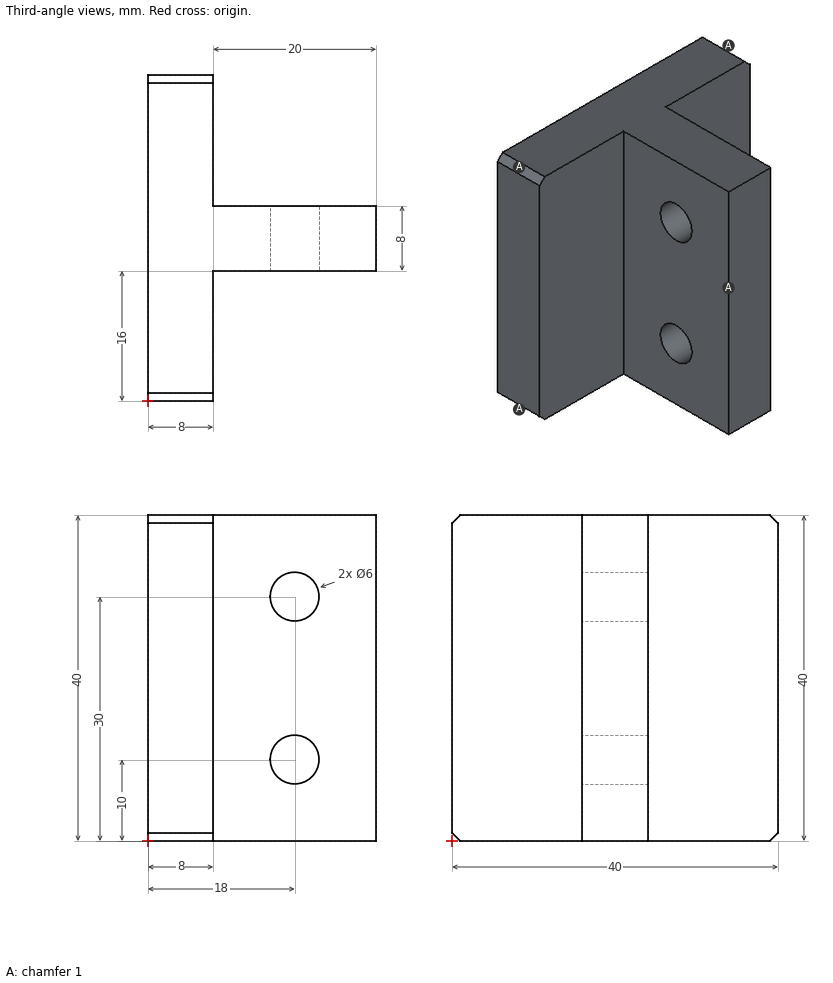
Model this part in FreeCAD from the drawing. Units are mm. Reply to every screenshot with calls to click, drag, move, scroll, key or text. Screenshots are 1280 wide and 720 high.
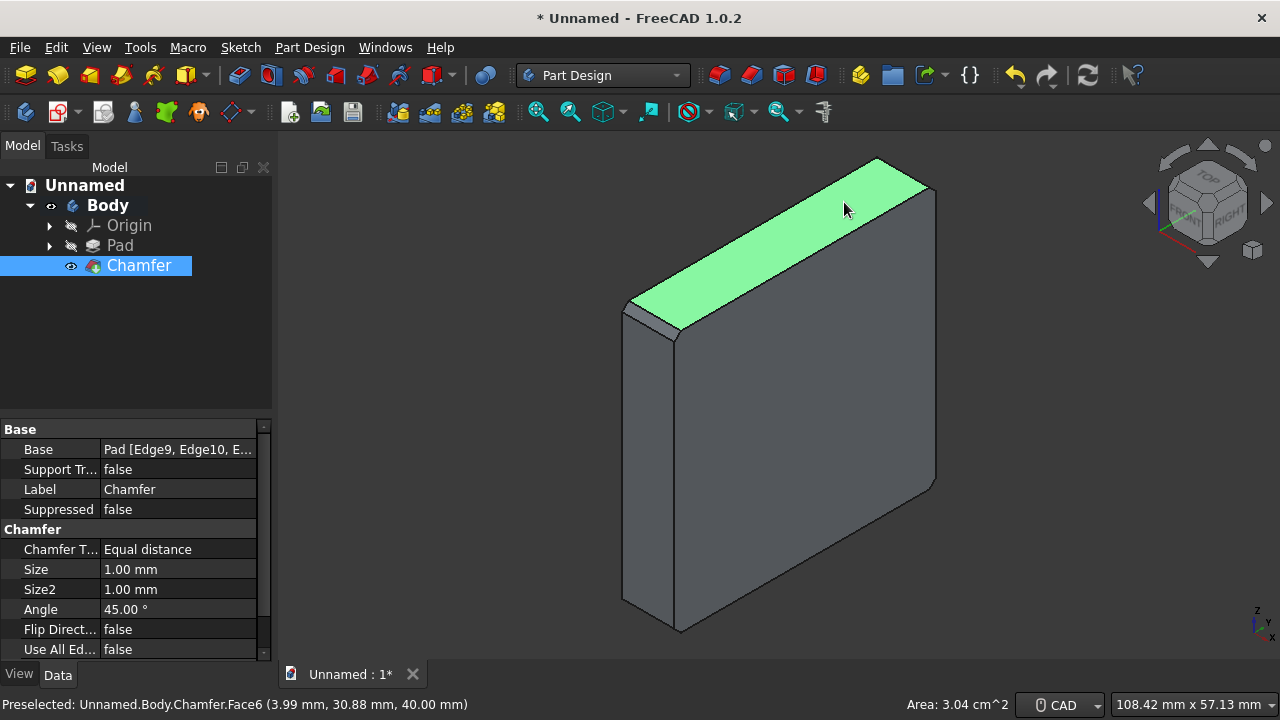
click(58, 112)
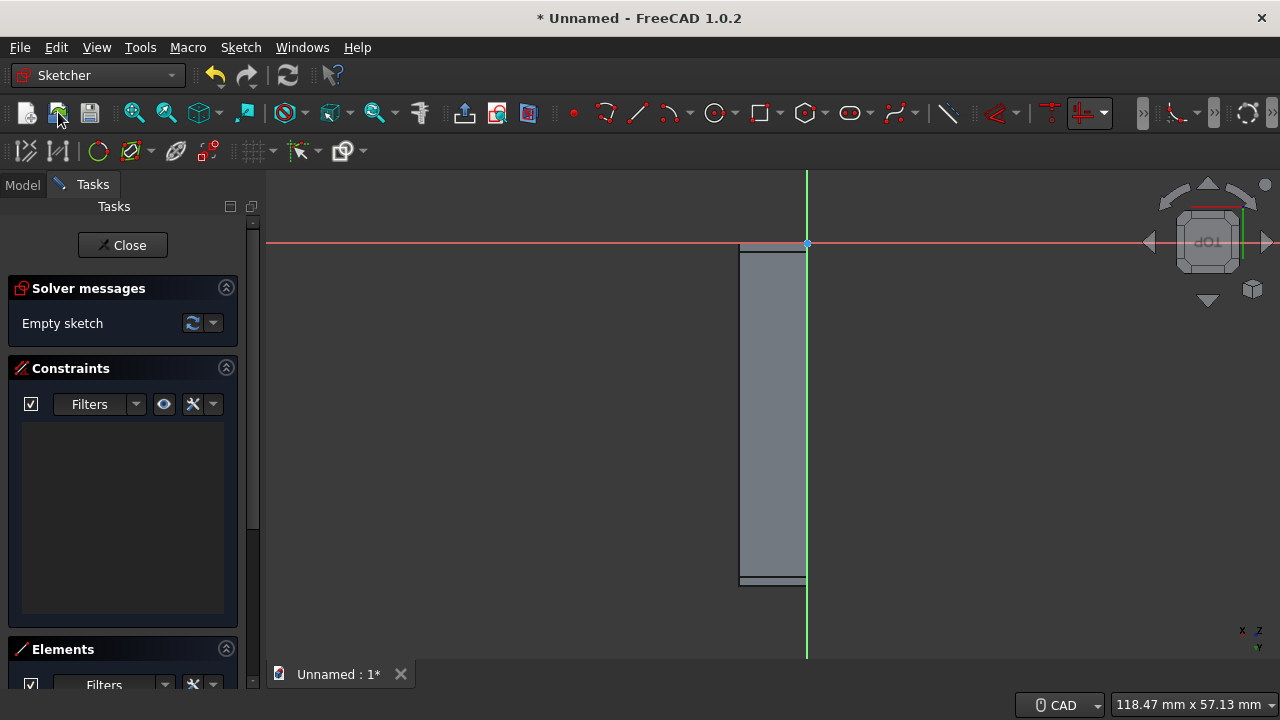
scroll(653, 207, up, 2)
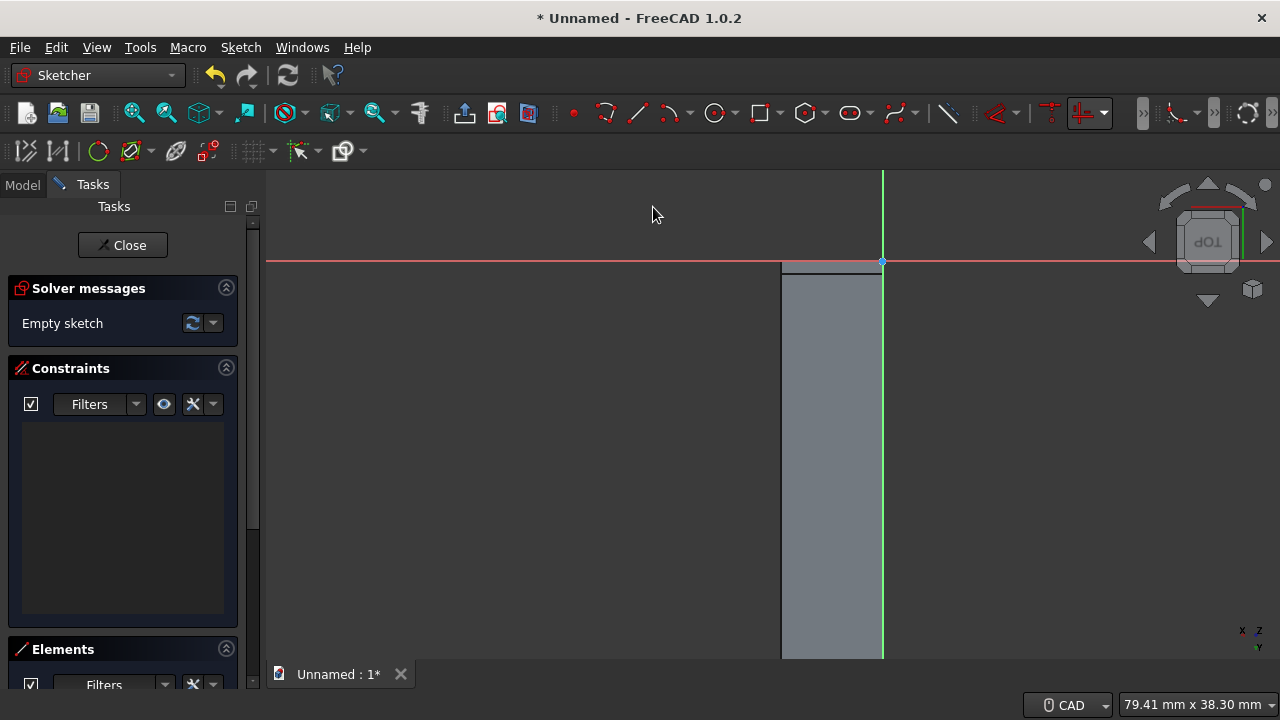
click(760, 114)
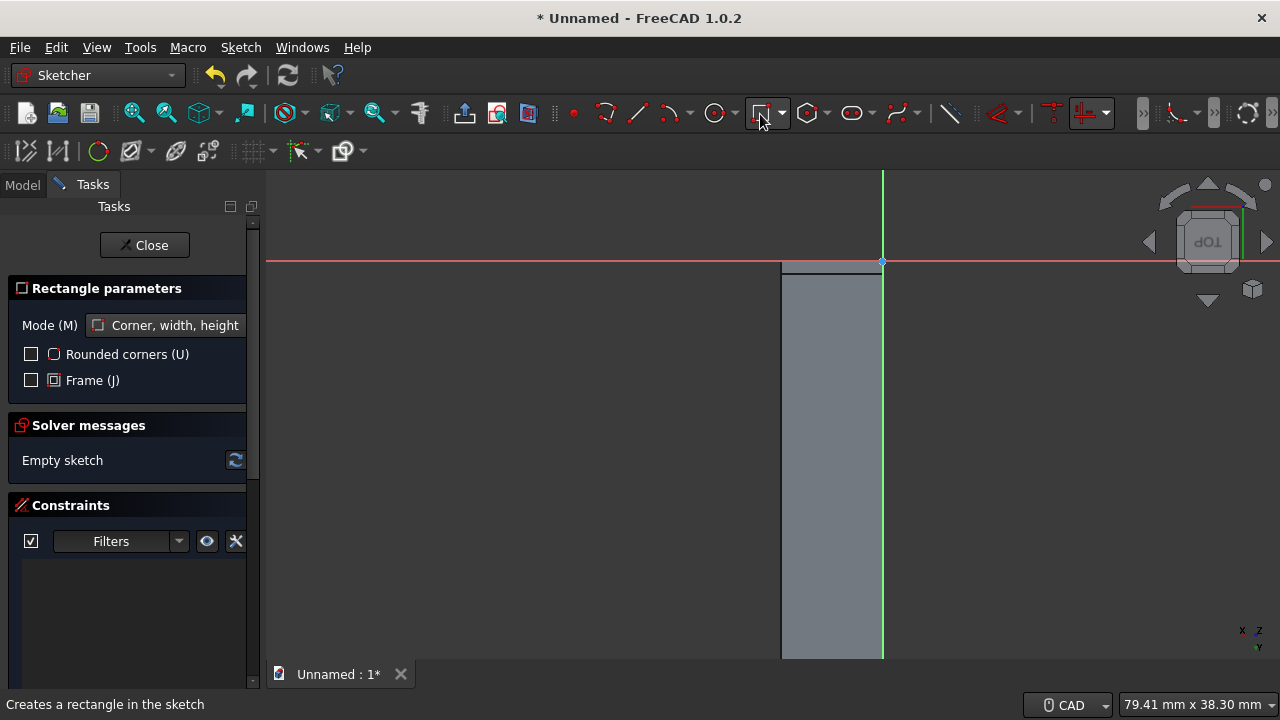
click(525, 465)
click(781, 568)
key(Escape)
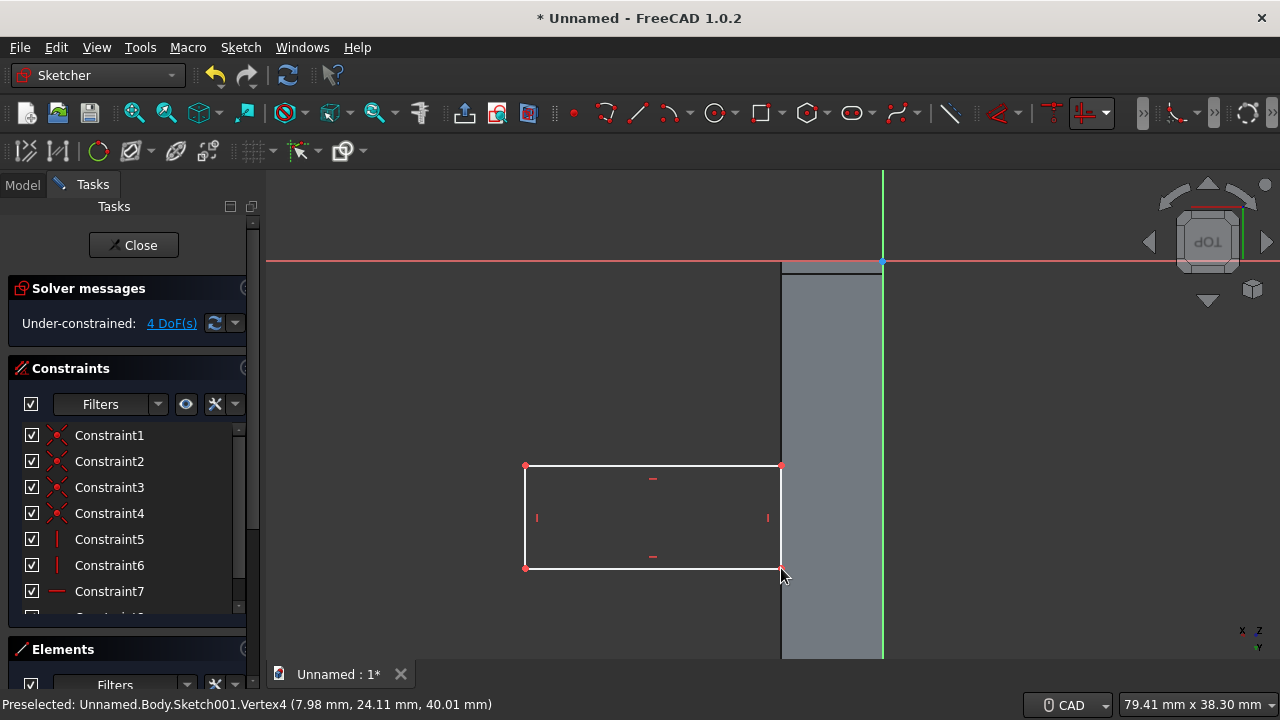
click(998, 114)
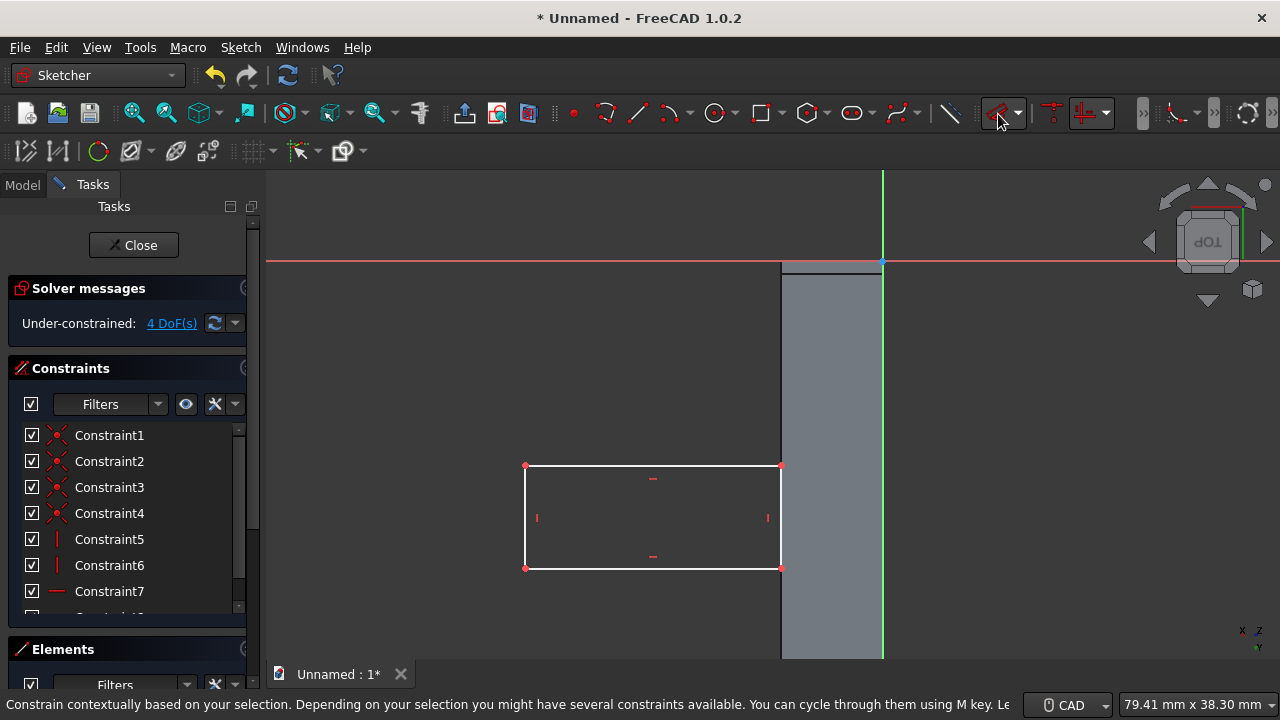
click(525, 497)
click(491, 518)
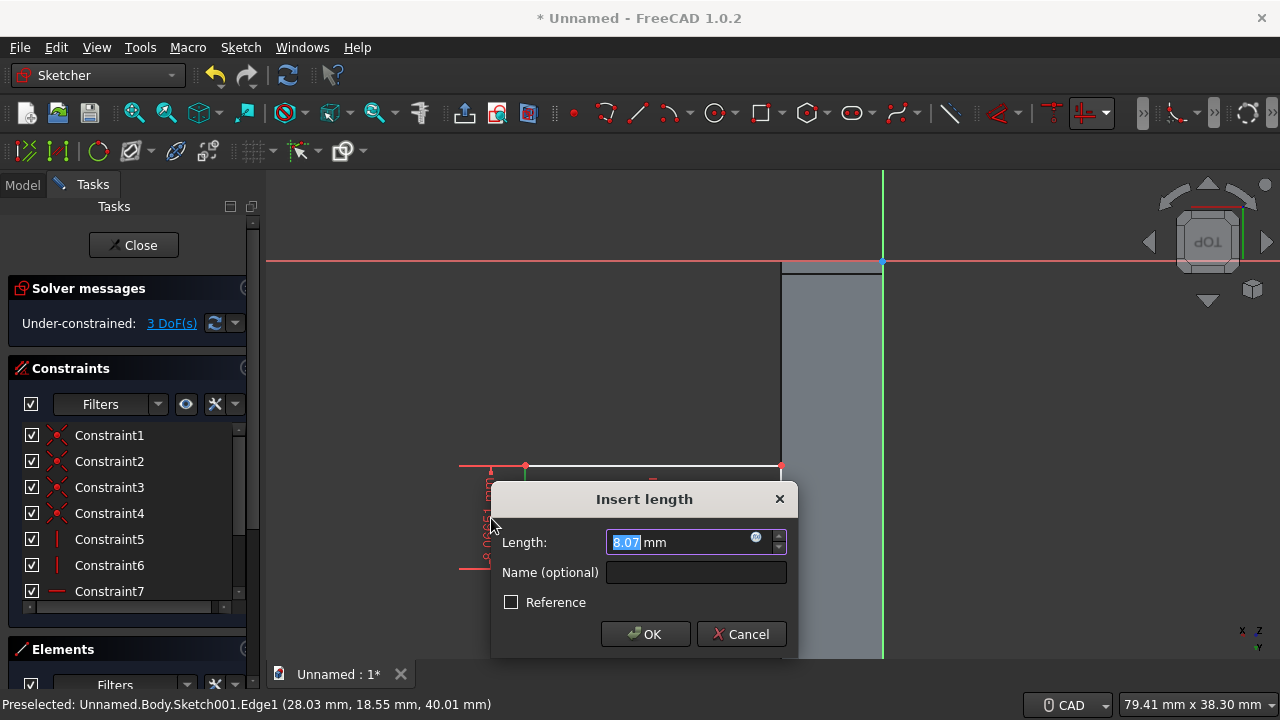
text(8)
key(Return)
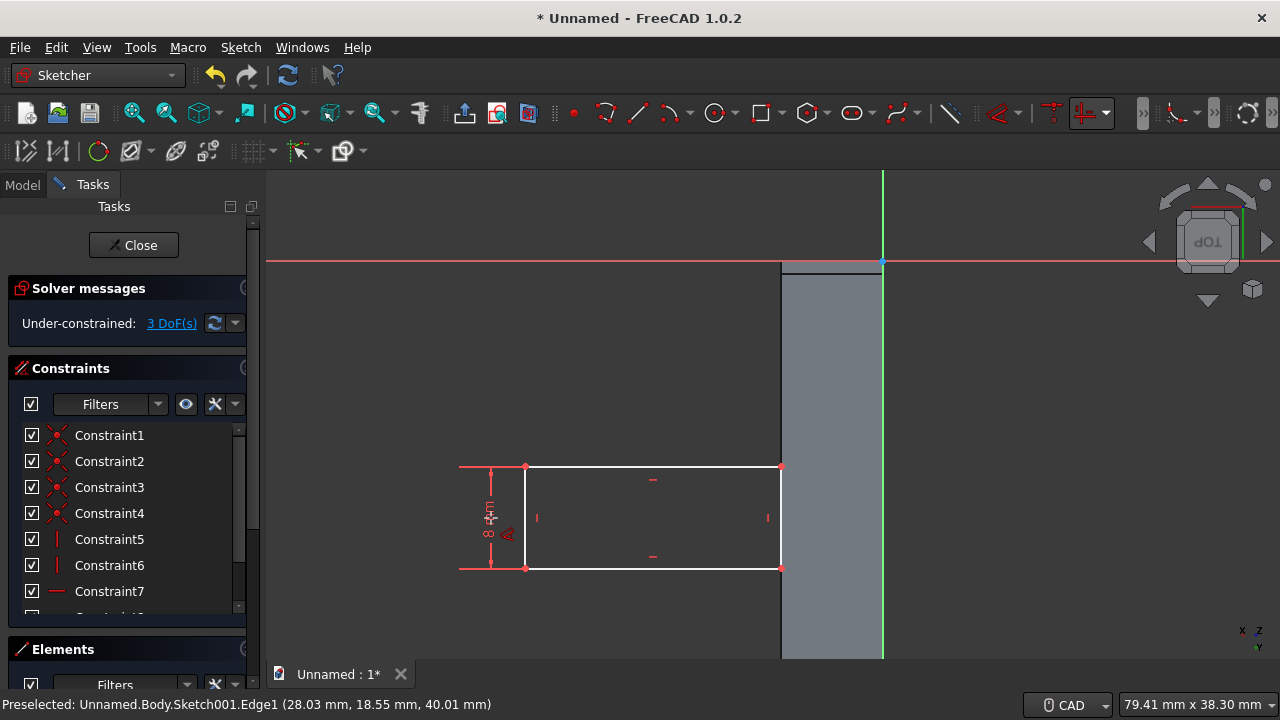
click(602, 569)
click(653, 603)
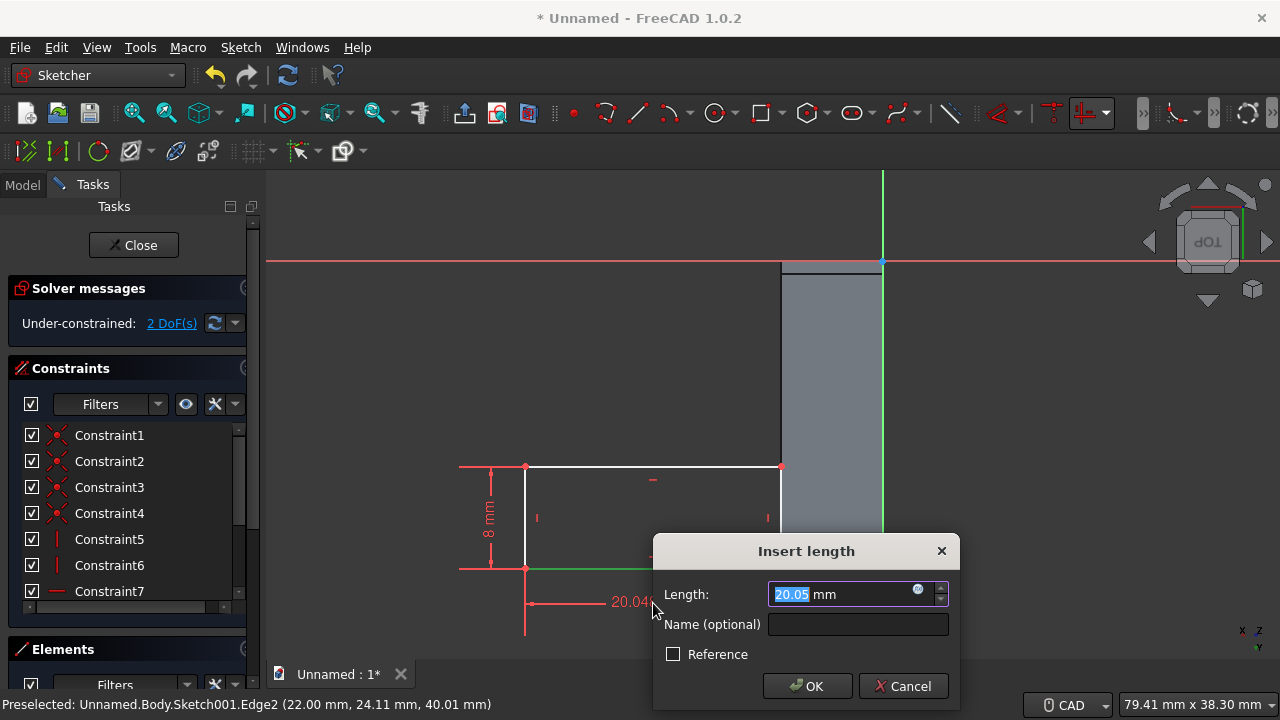
text(20)
key(Return)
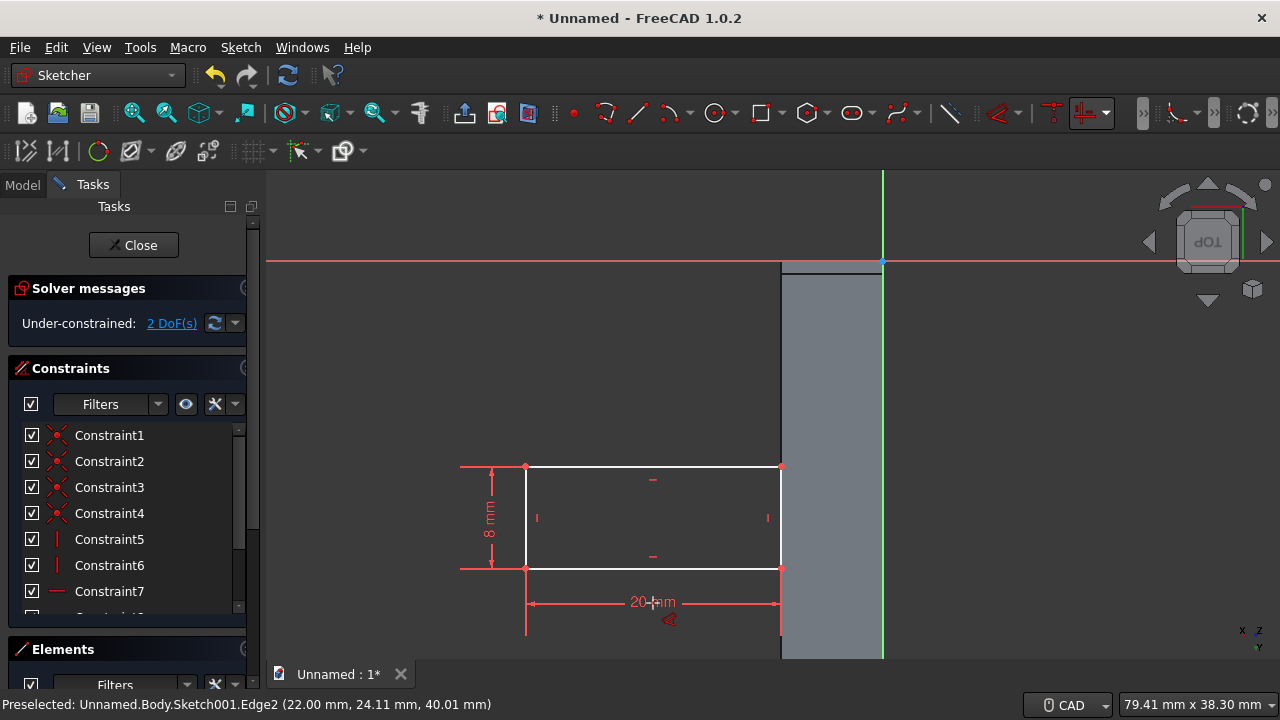
click(781, 569)
click(832, 603)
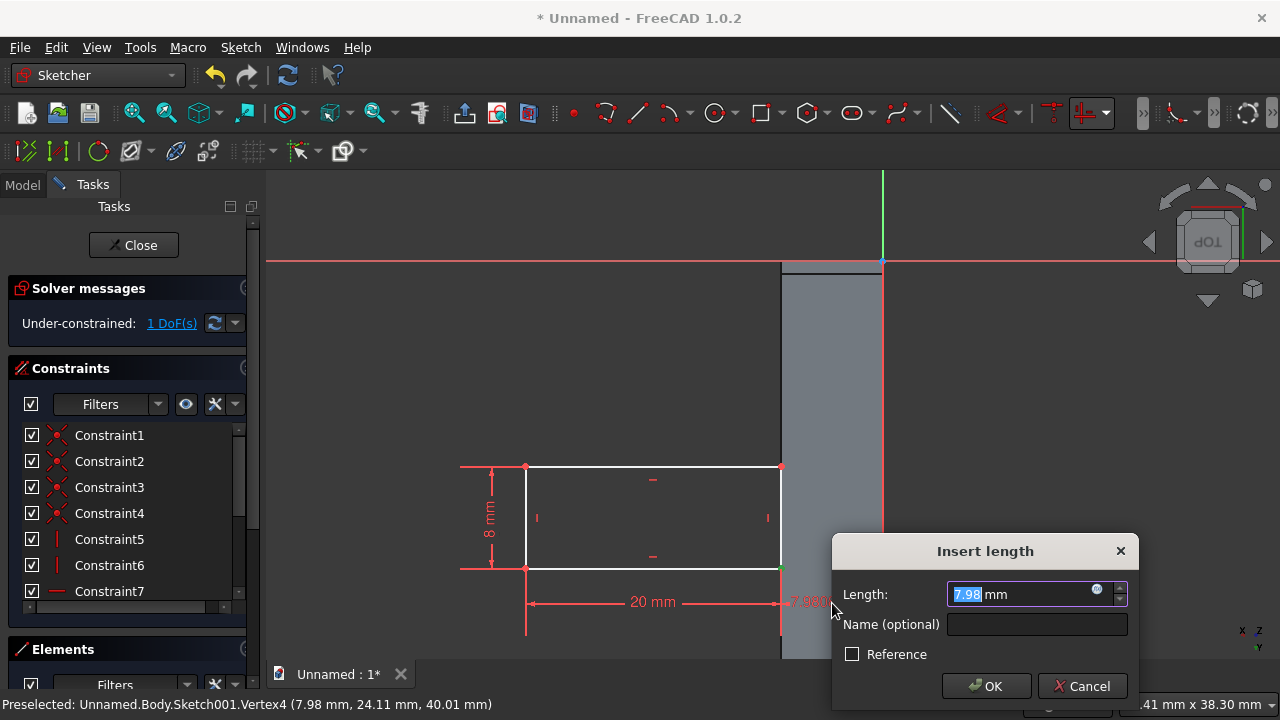
text(8)
key(Return)